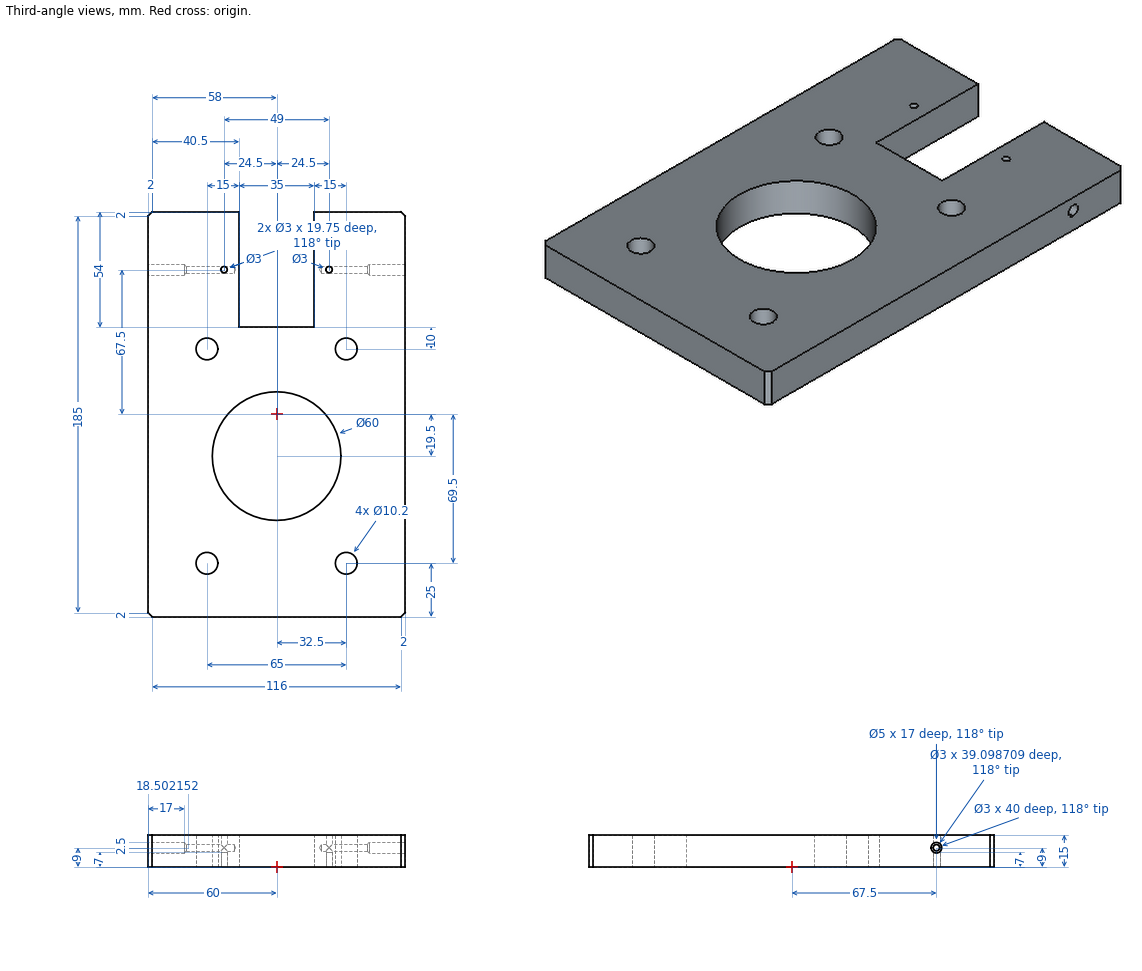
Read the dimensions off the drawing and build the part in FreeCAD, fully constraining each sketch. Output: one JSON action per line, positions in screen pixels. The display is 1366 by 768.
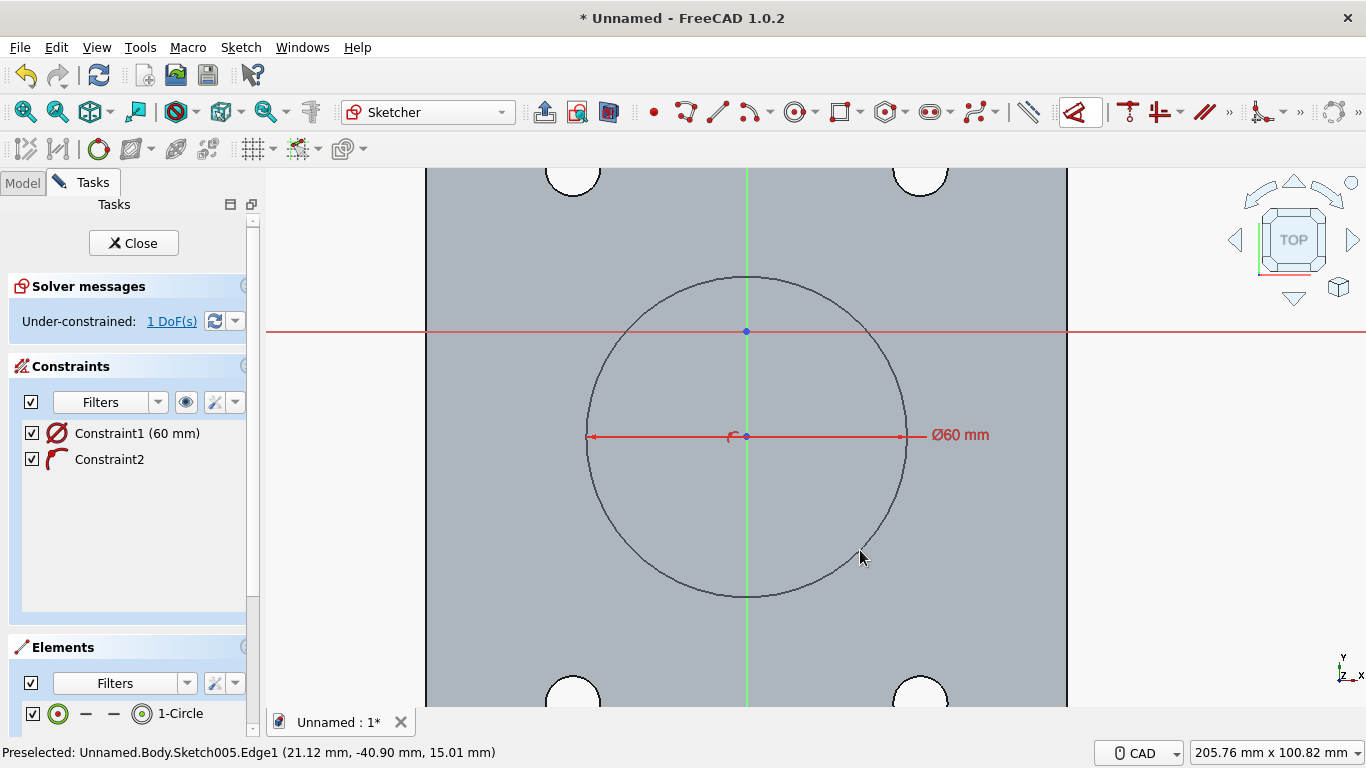
{"action": "left_click", "coordinate": [747, 437]}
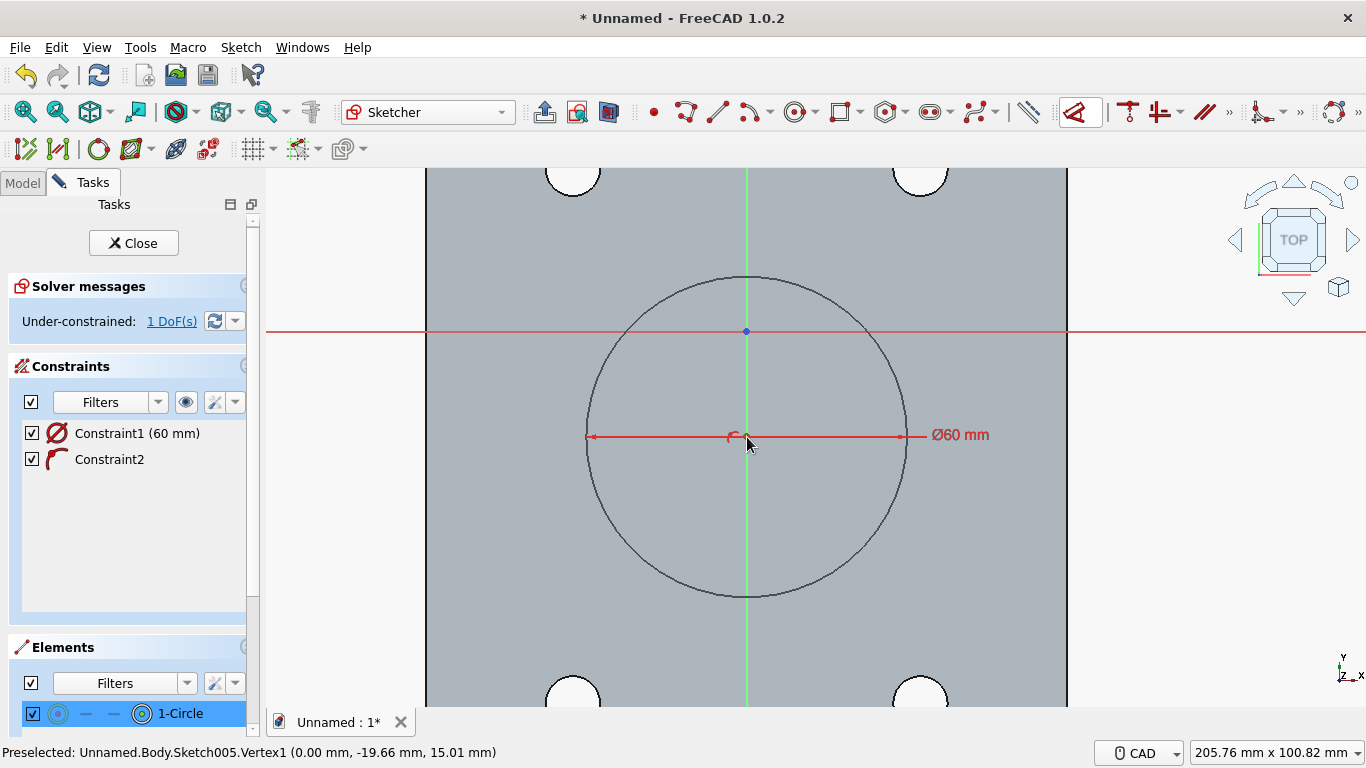
{"action": "left_click", "coordinate": [1096, 112]}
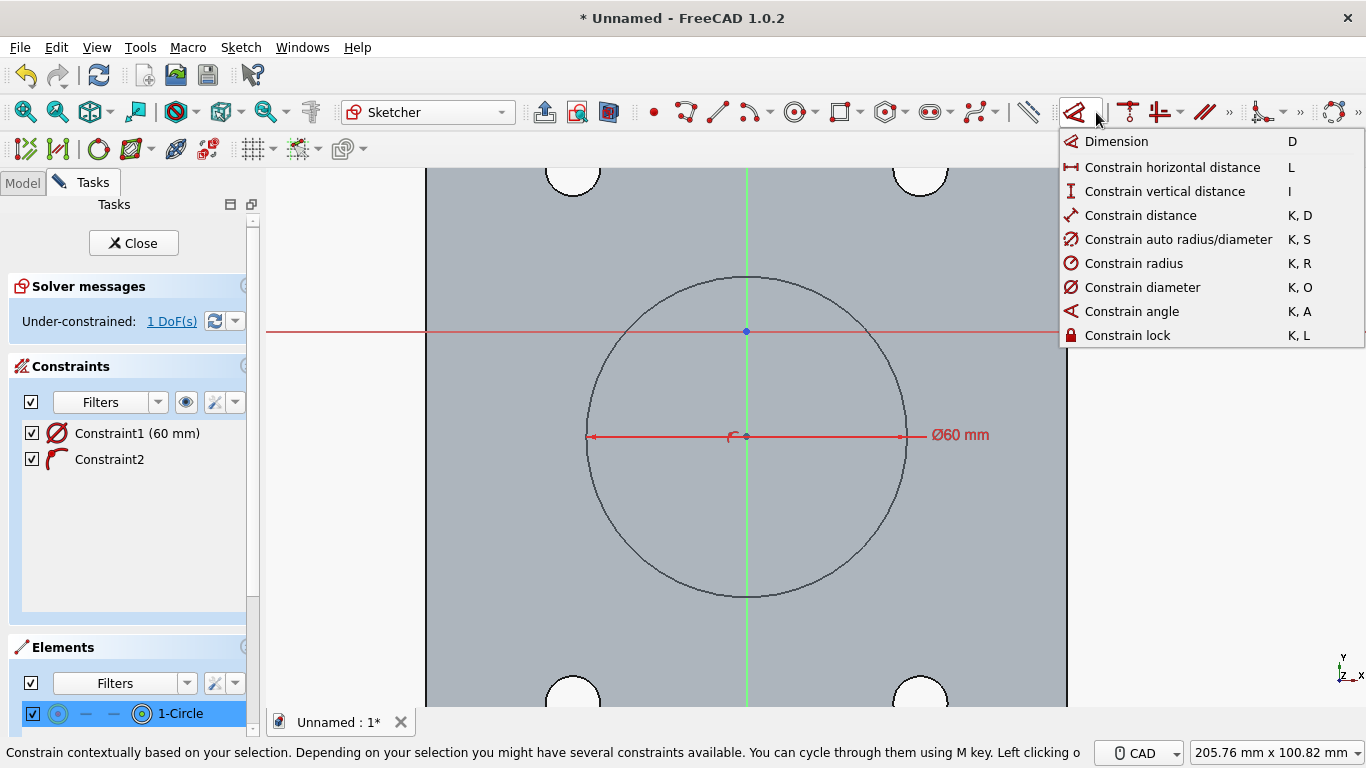
{"action": "left_click", "coordinate": [1212, 191]}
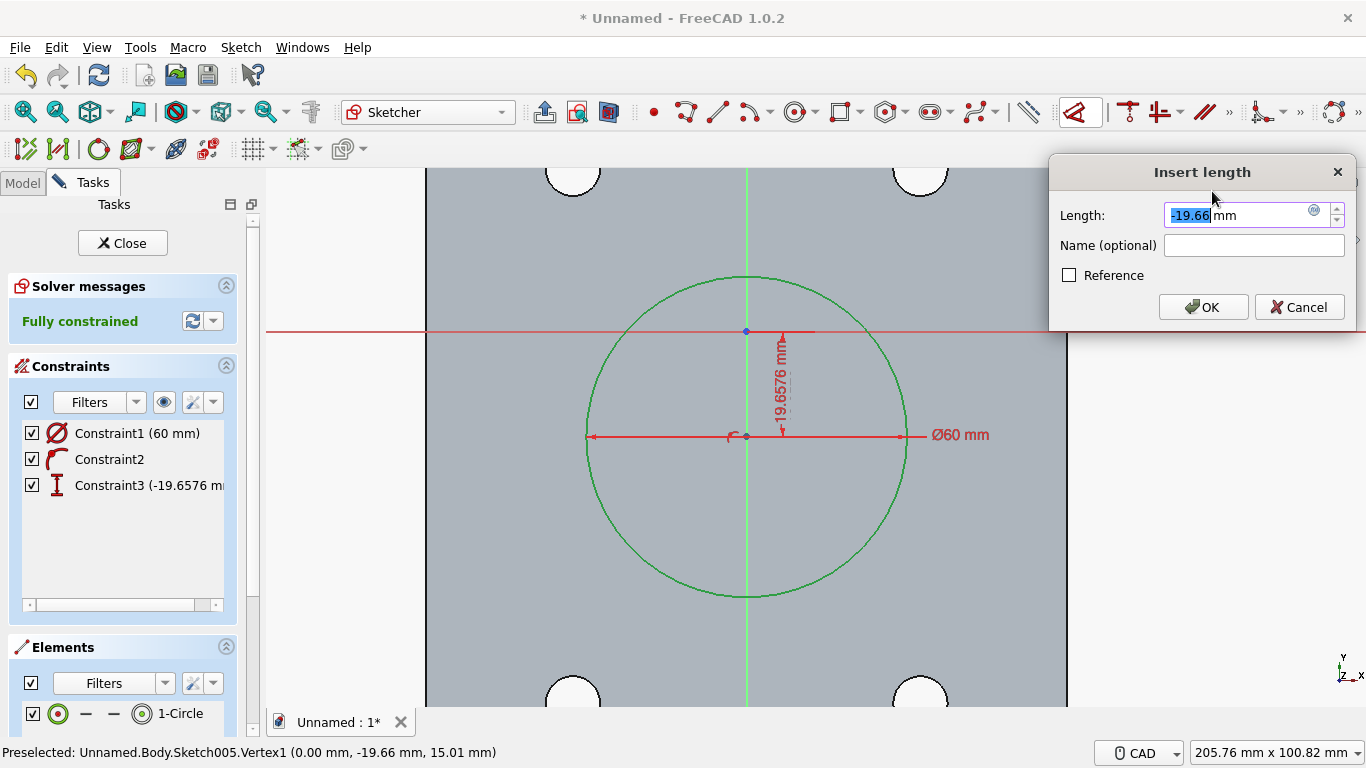
{"action": "type", "text": "-19.5"}
{"action": "key", "text": "Return"}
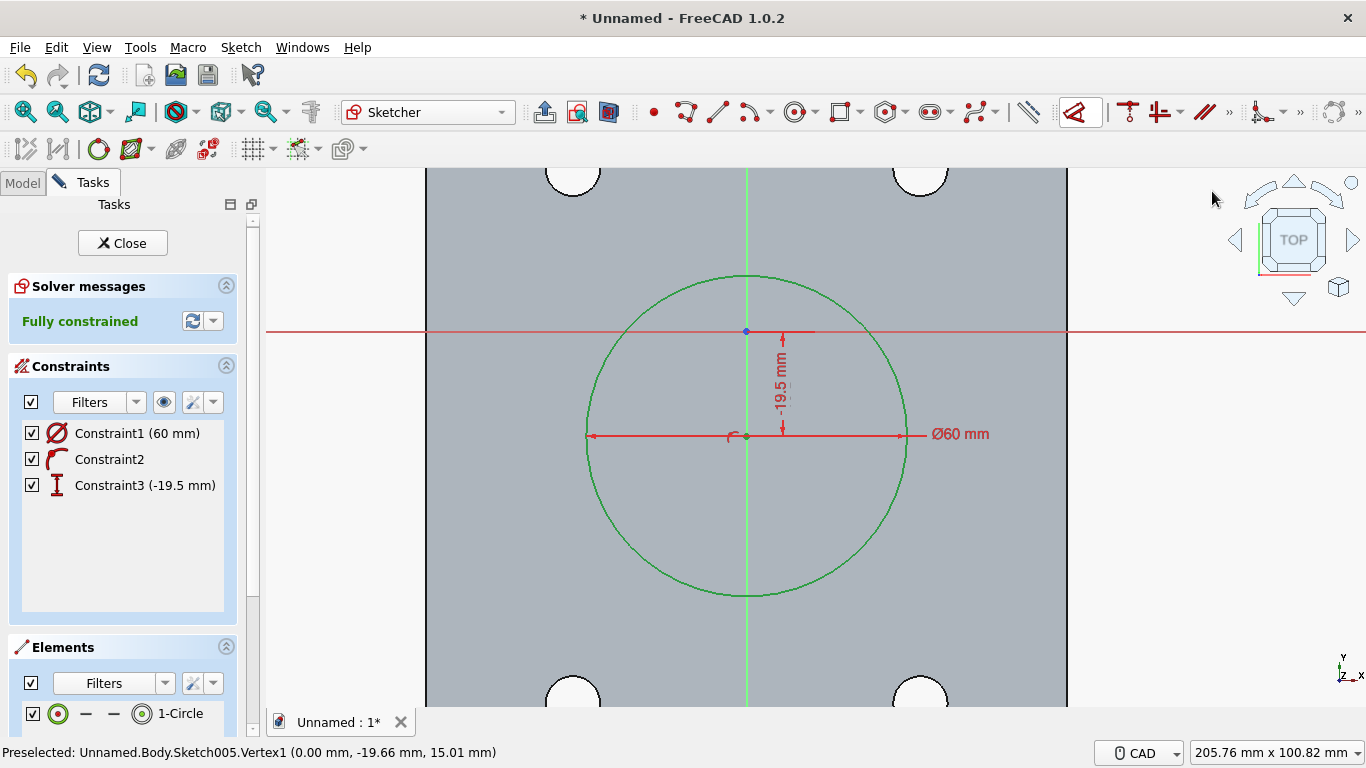
{"action": "left_click", "coordinate": [123, 243]}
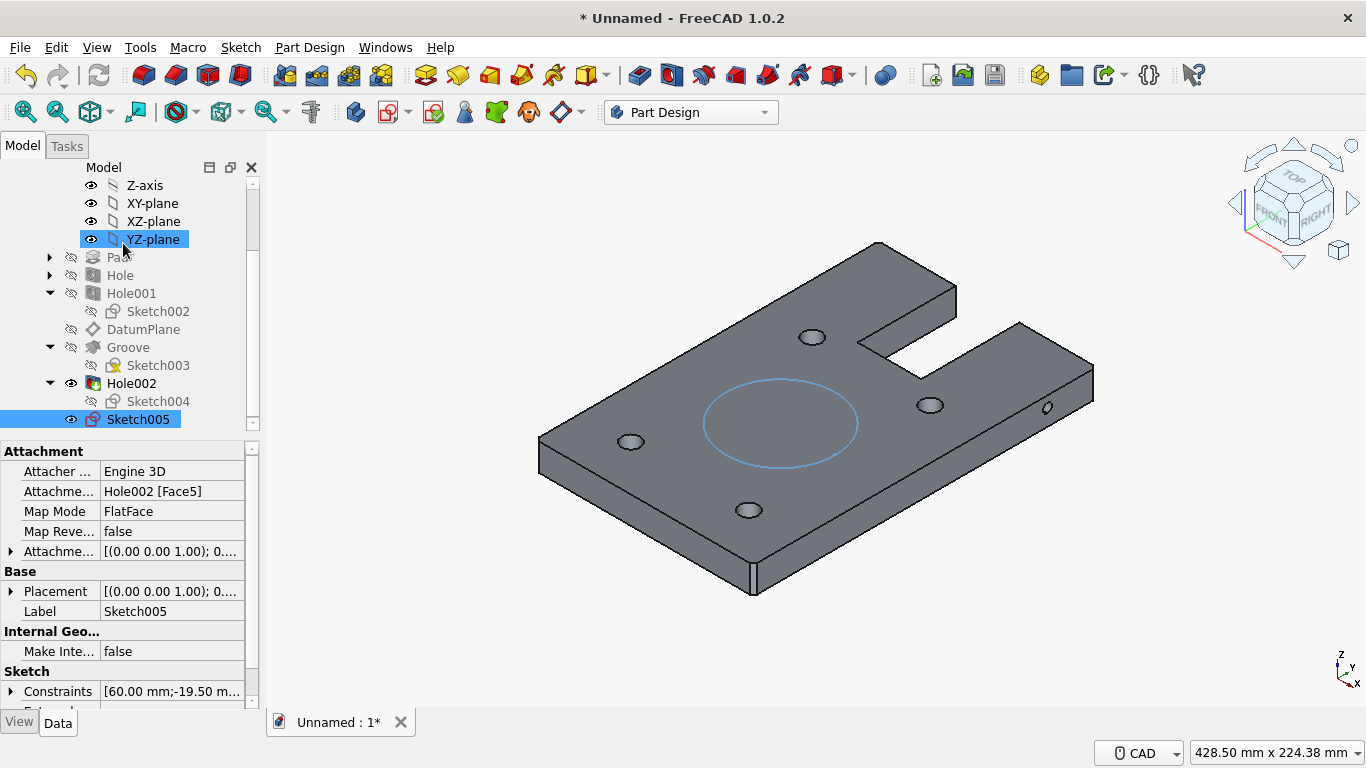
{"action": "left_click", "coordinate": [640, 76]}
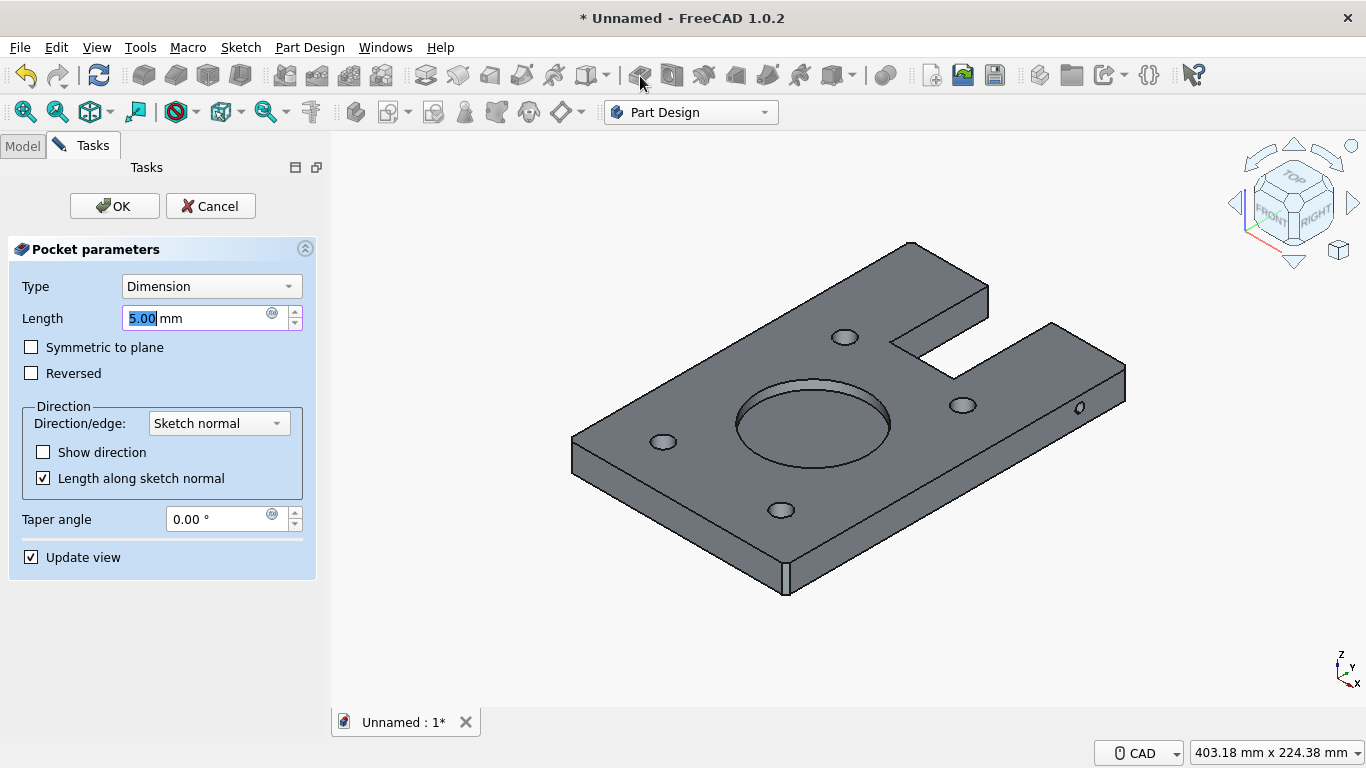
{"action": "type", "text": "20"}
{"action": "key", "text": "Tab"}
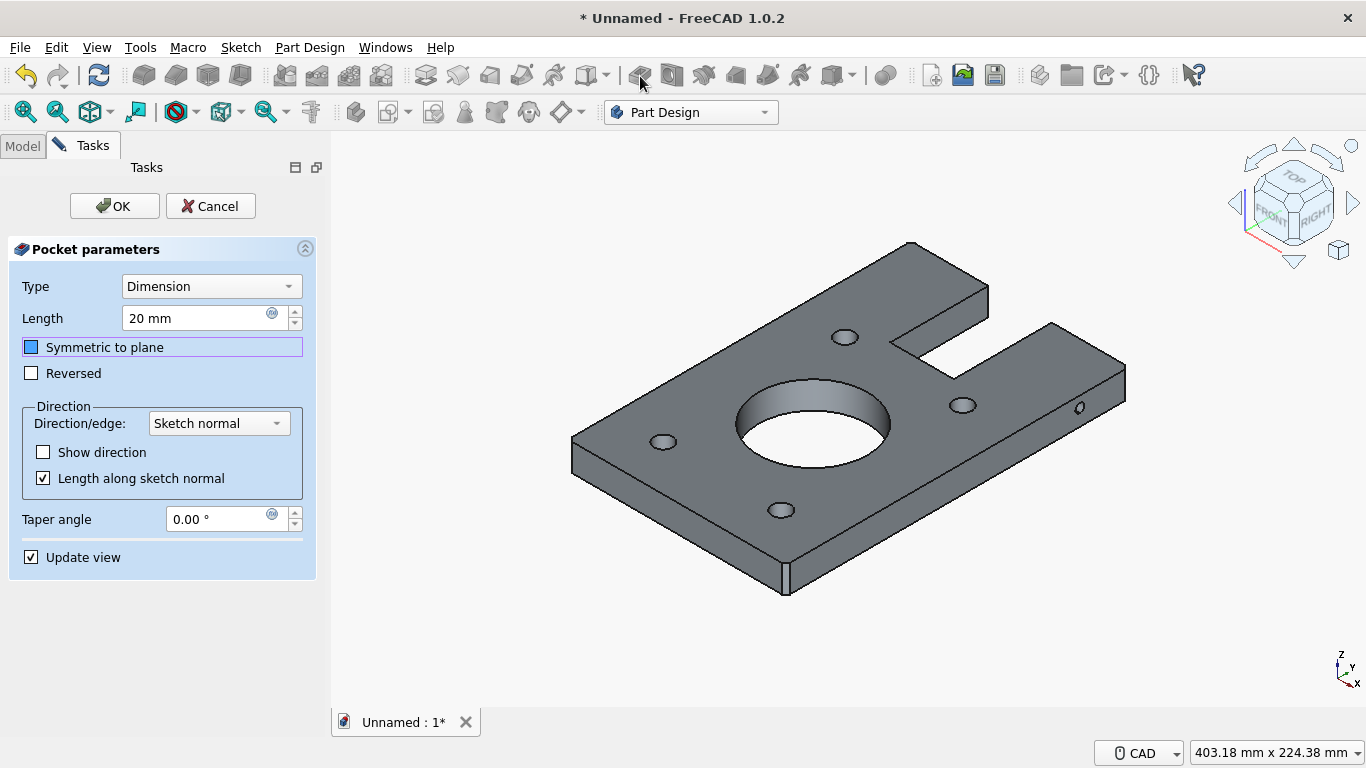
{"action": "left_click", "coordinate": [115, 206]}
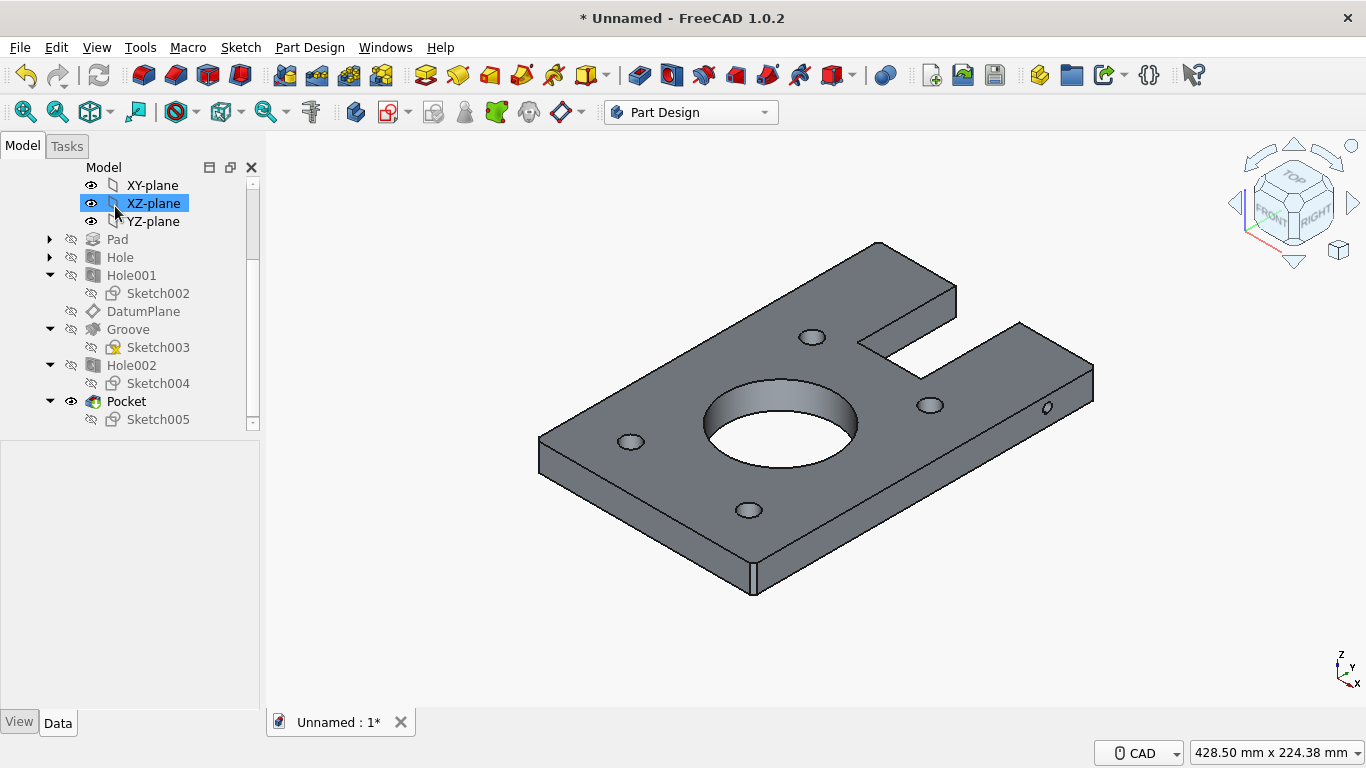
{"action": "left_click", "coordinate": [976, 382]}